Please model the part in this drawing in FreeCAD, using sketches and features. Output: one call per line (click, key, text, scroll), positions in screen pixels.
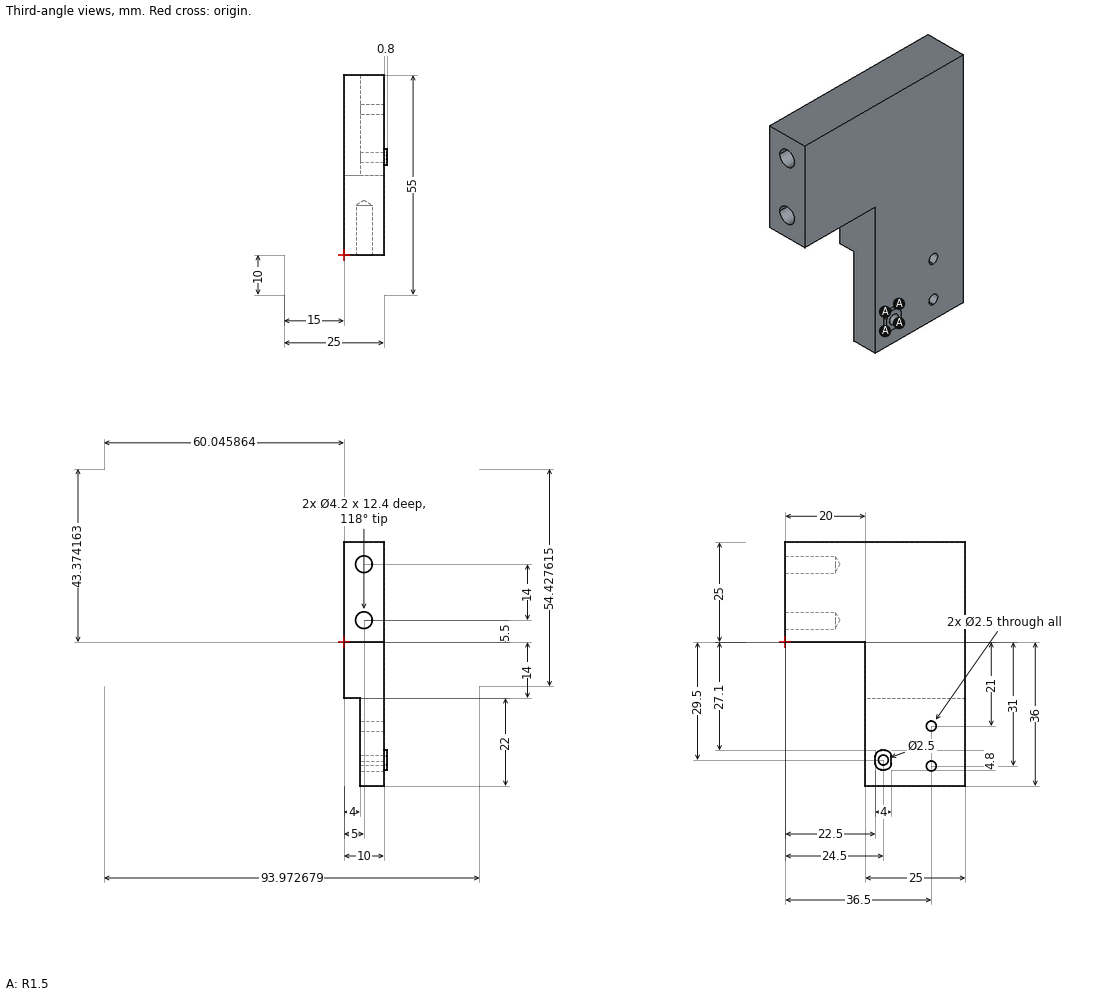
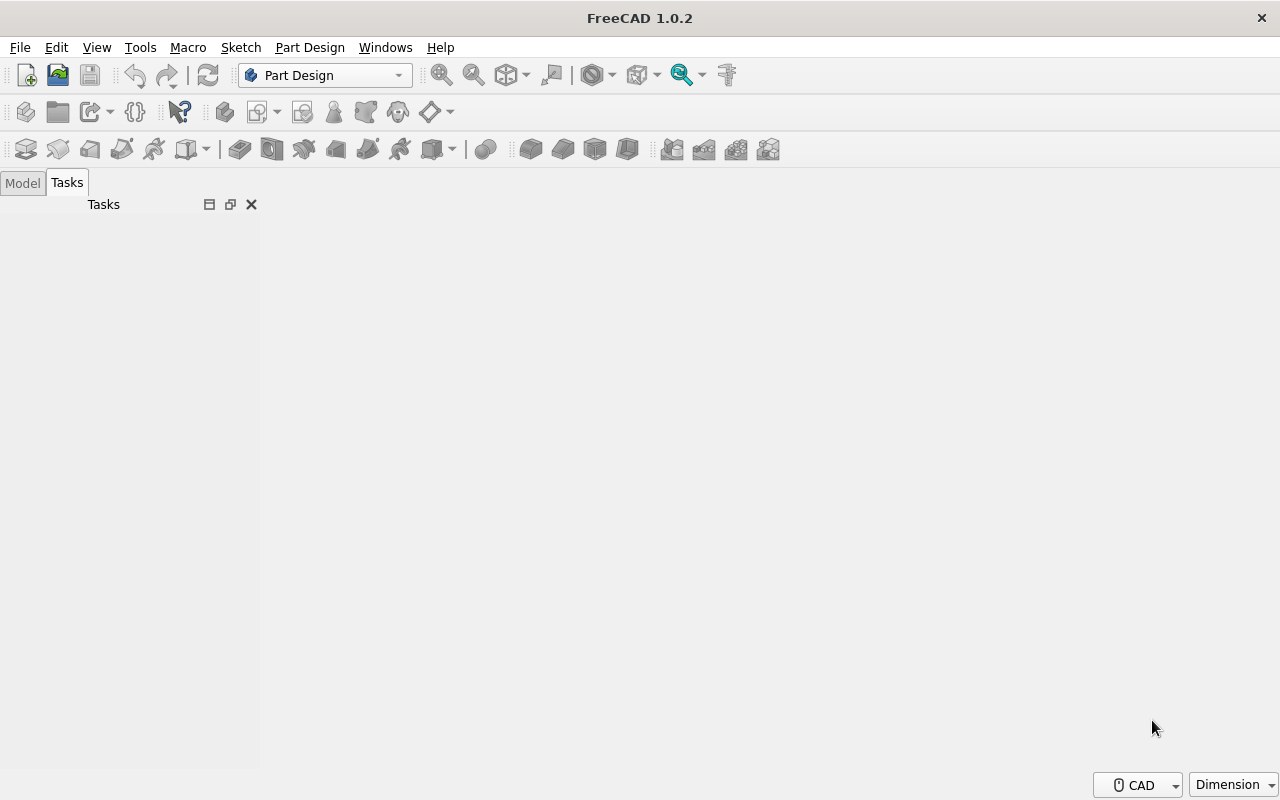
click(26, 76)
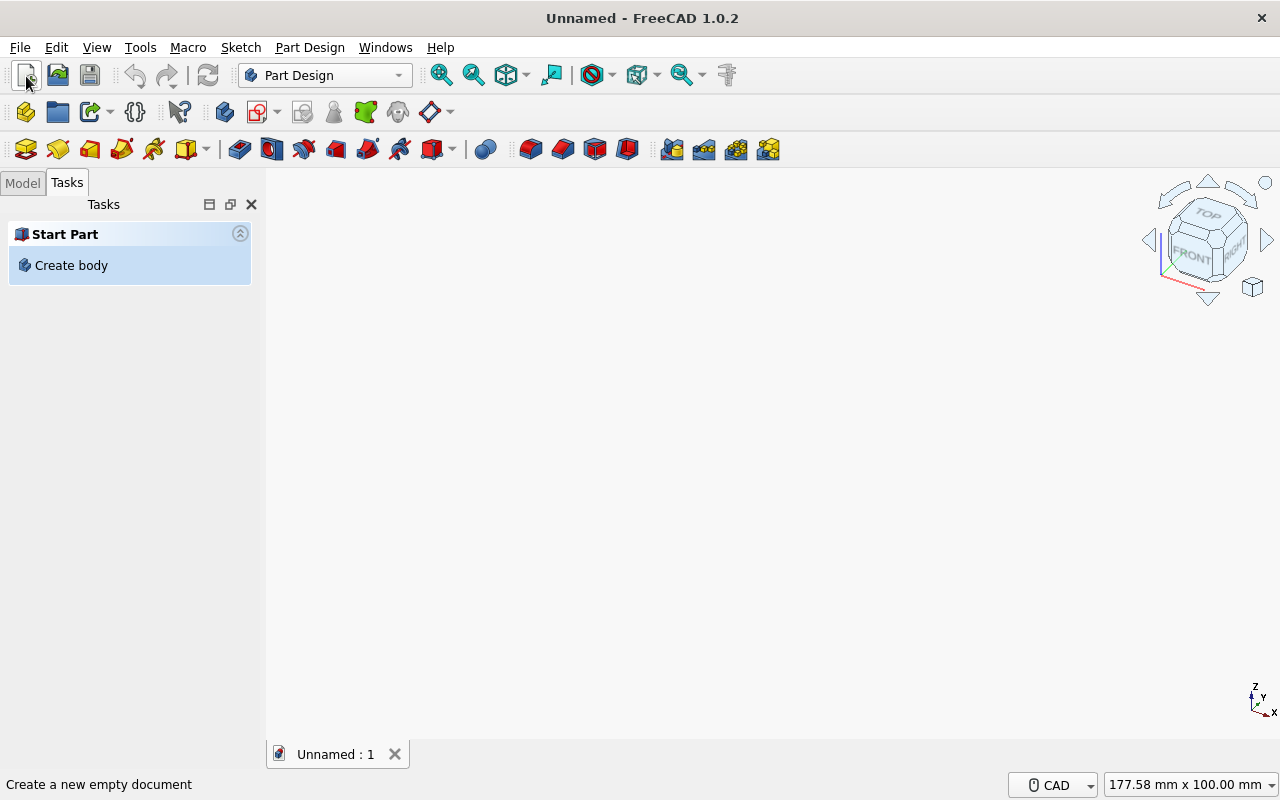
click(258, 112)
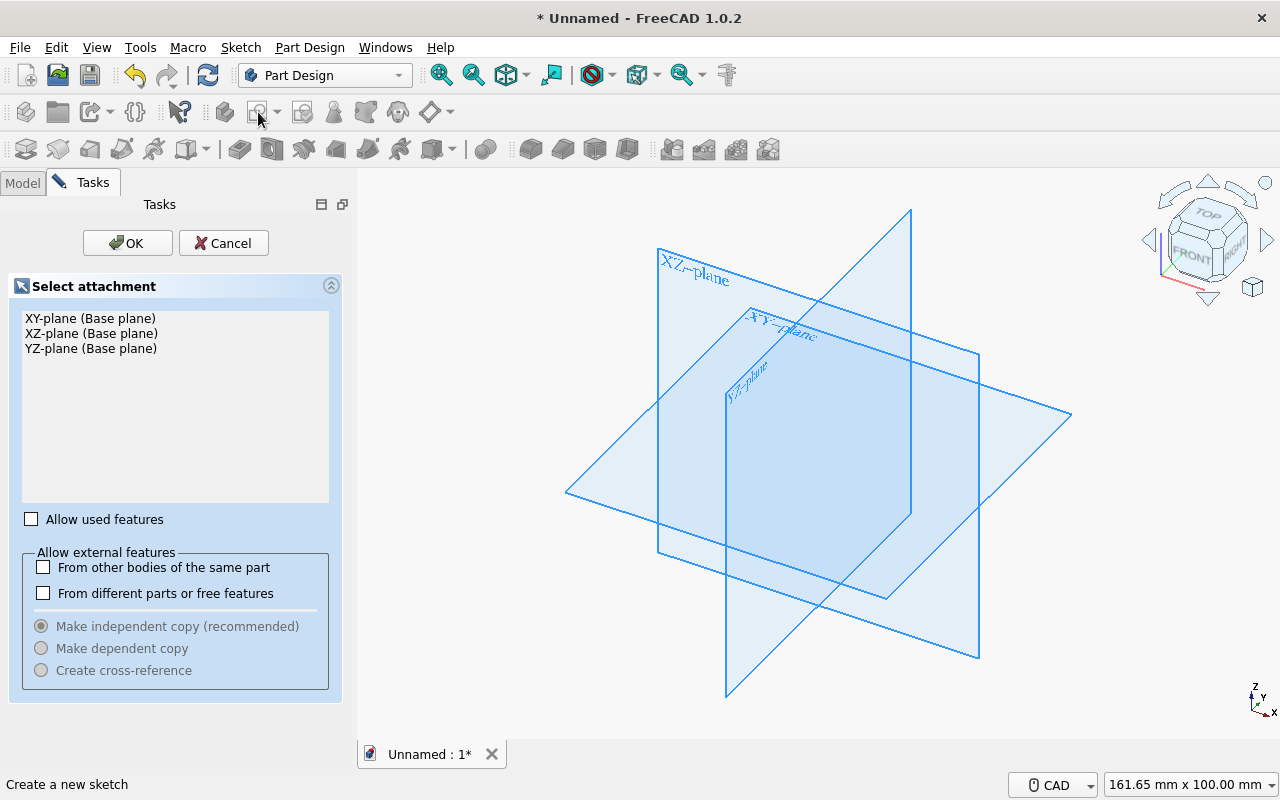
click(82, 318)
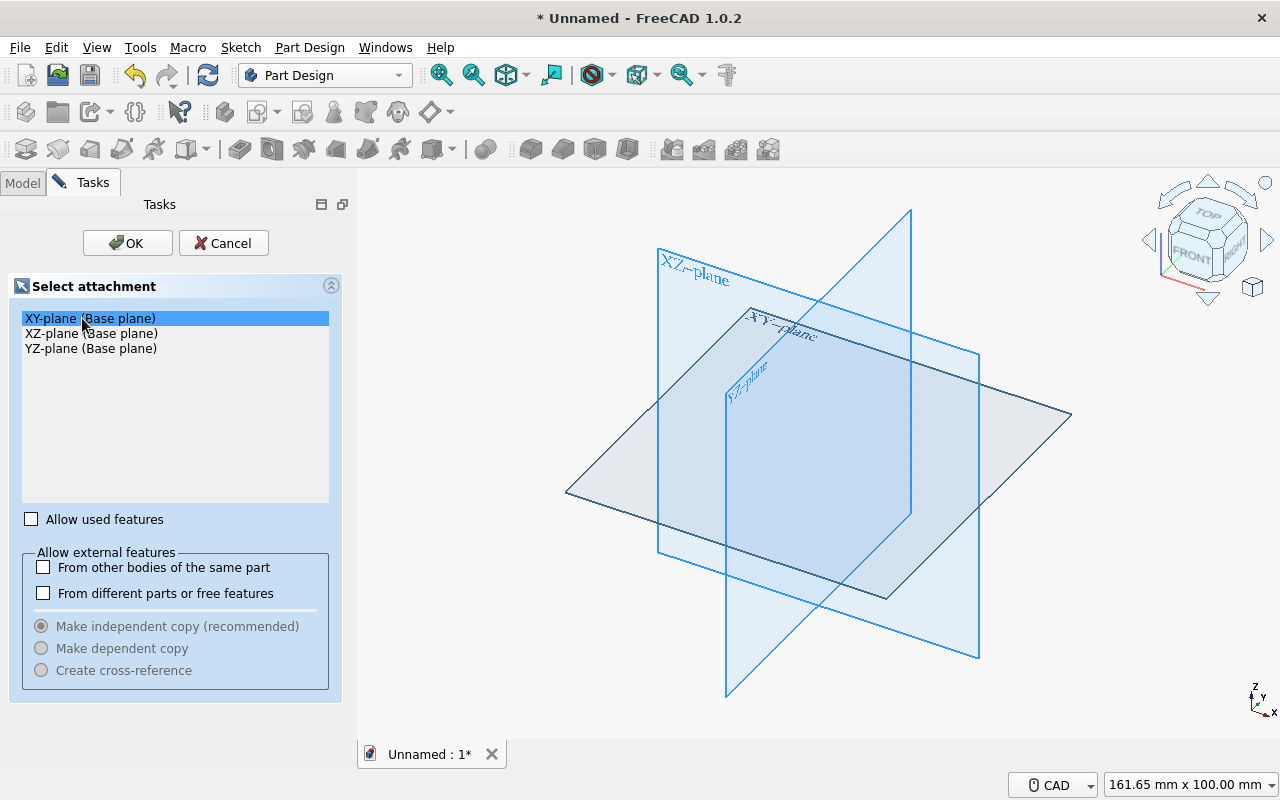
click(128, 243)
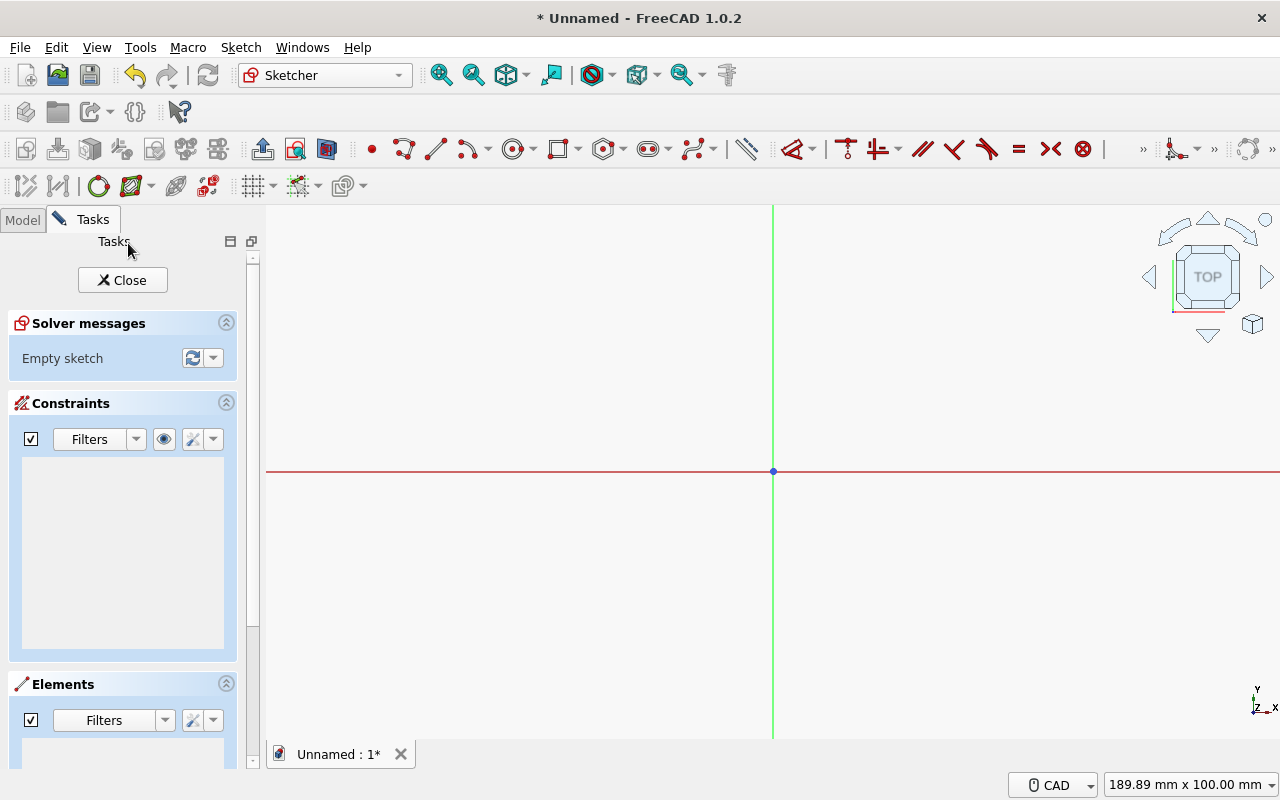
scroll(455, 711, down, 1)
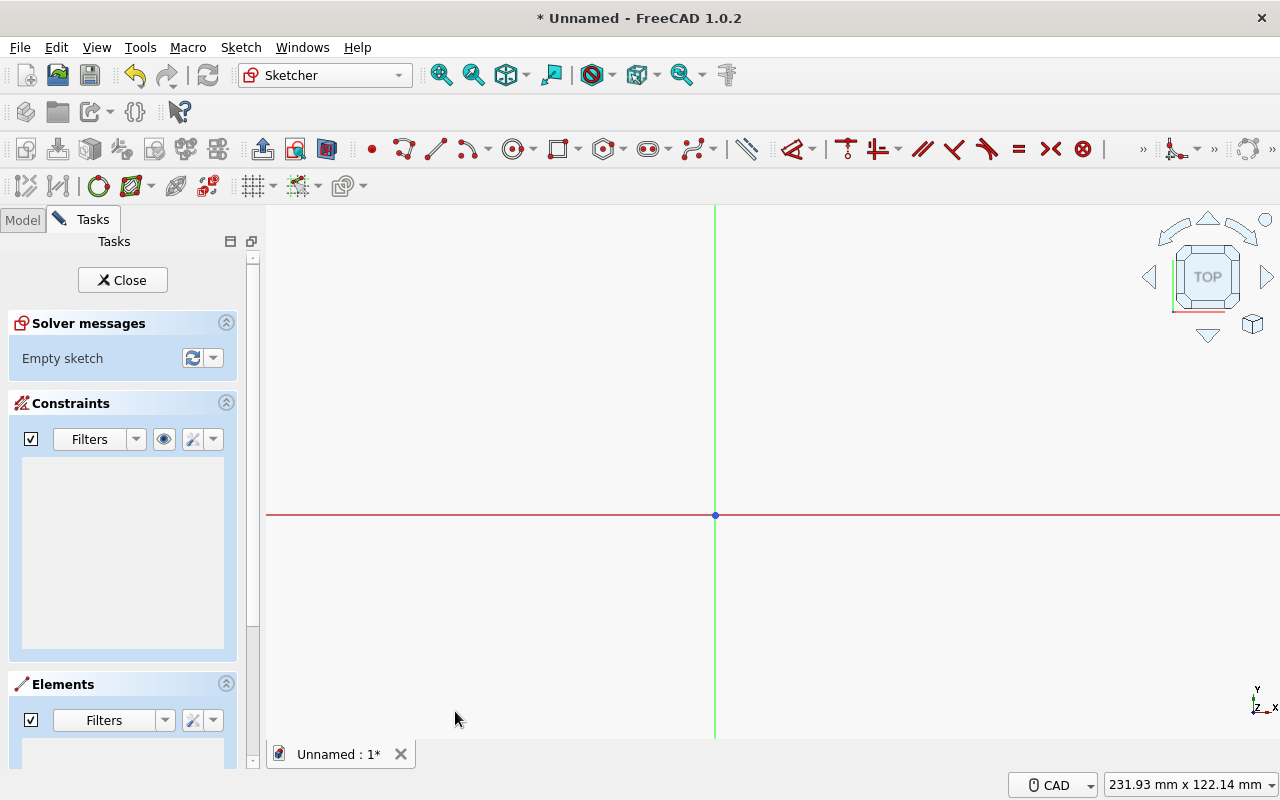
scroll(704, 372, up, 2)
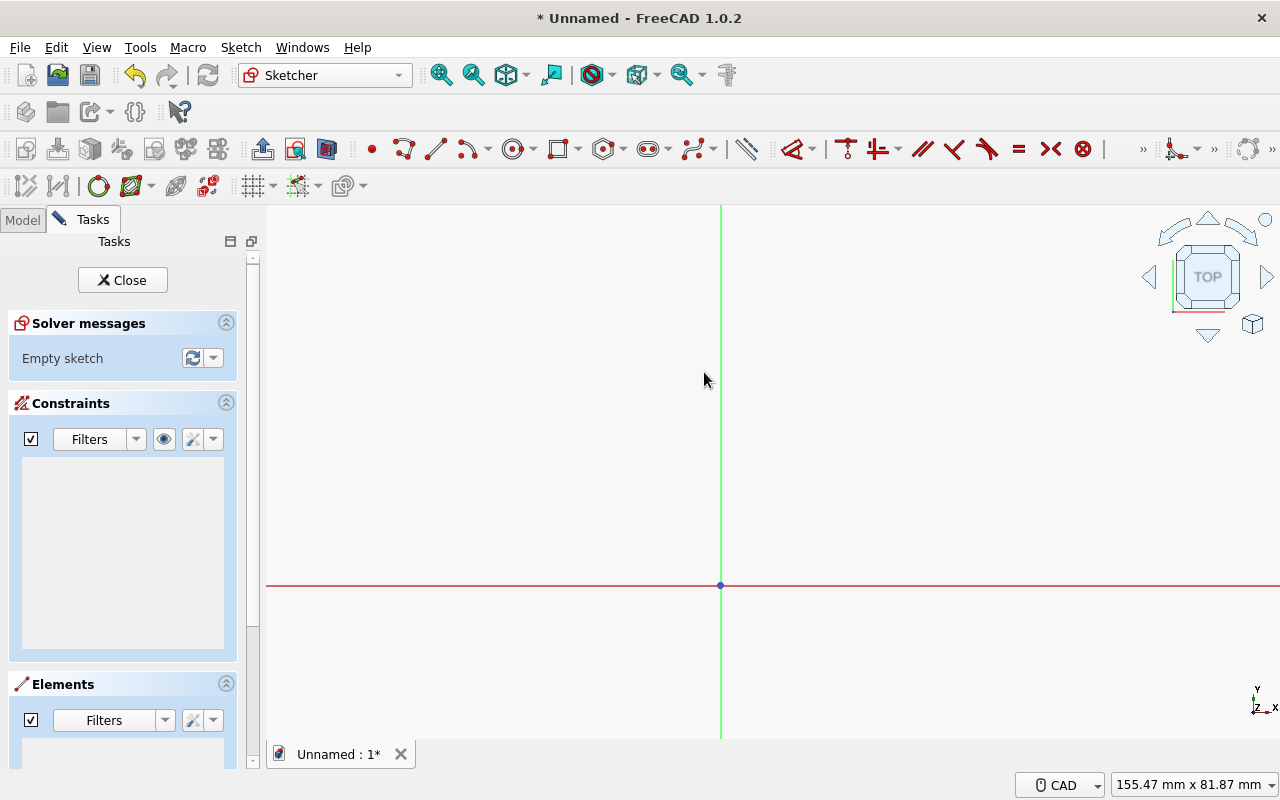
click(404, 150)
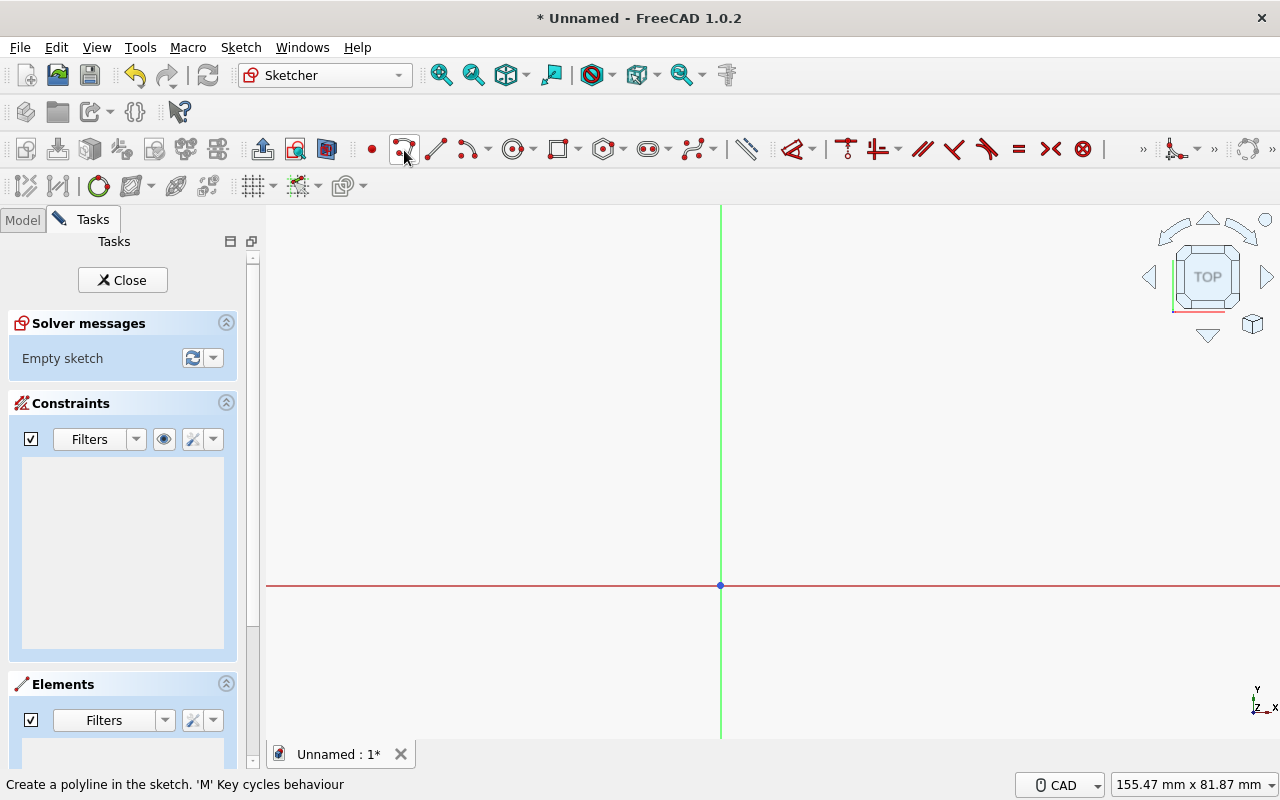
click(721, 586)
click(623, 577)
click(623, 651)
click(786, 651)
click(786, 292)
click(712, 292)
click(721, 586)
key(Escape)
key(Escape)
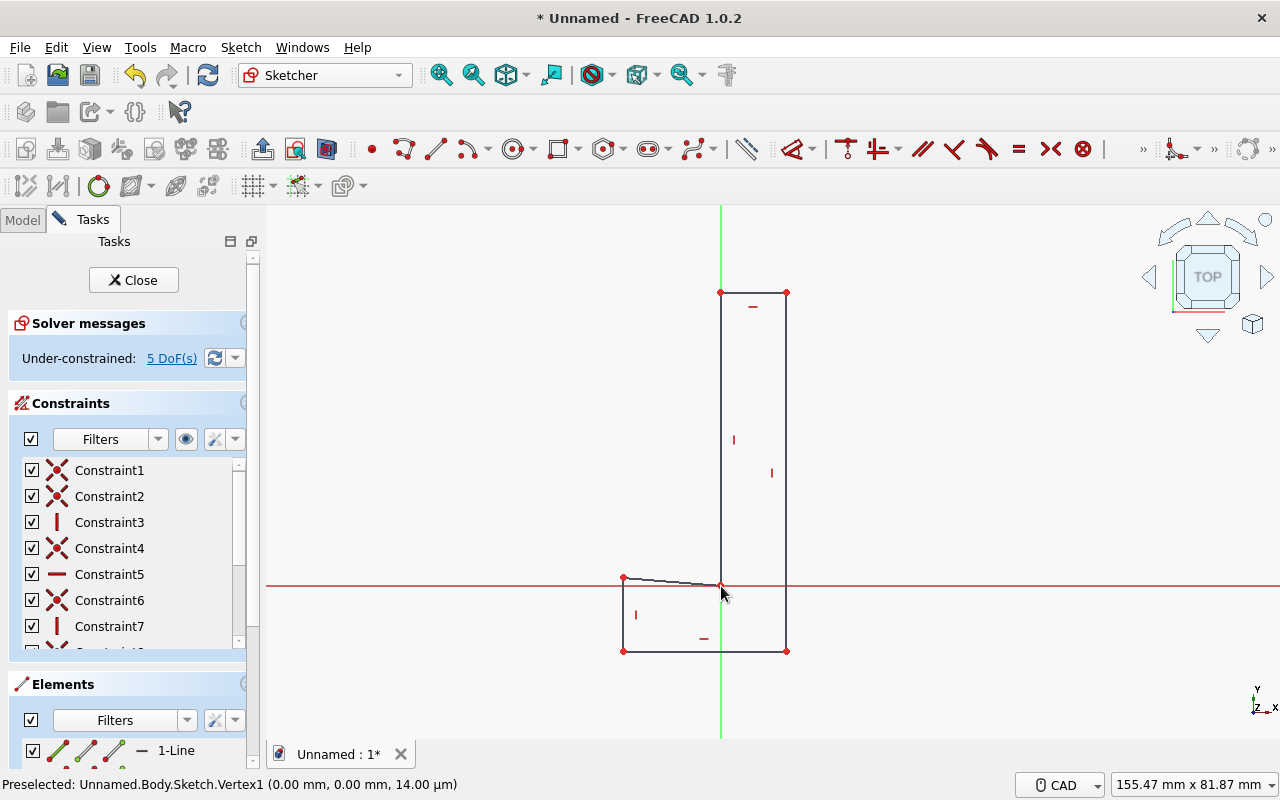
click(691, 584)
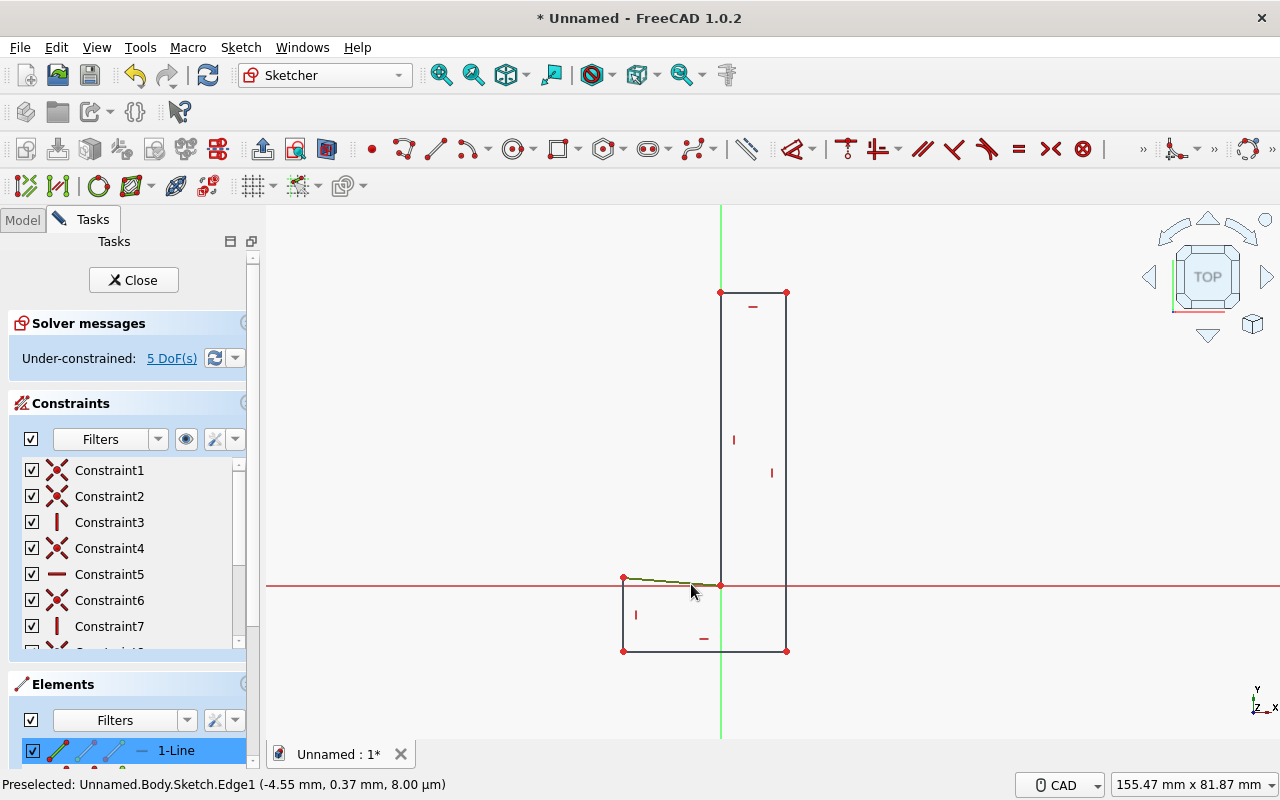
key(h)